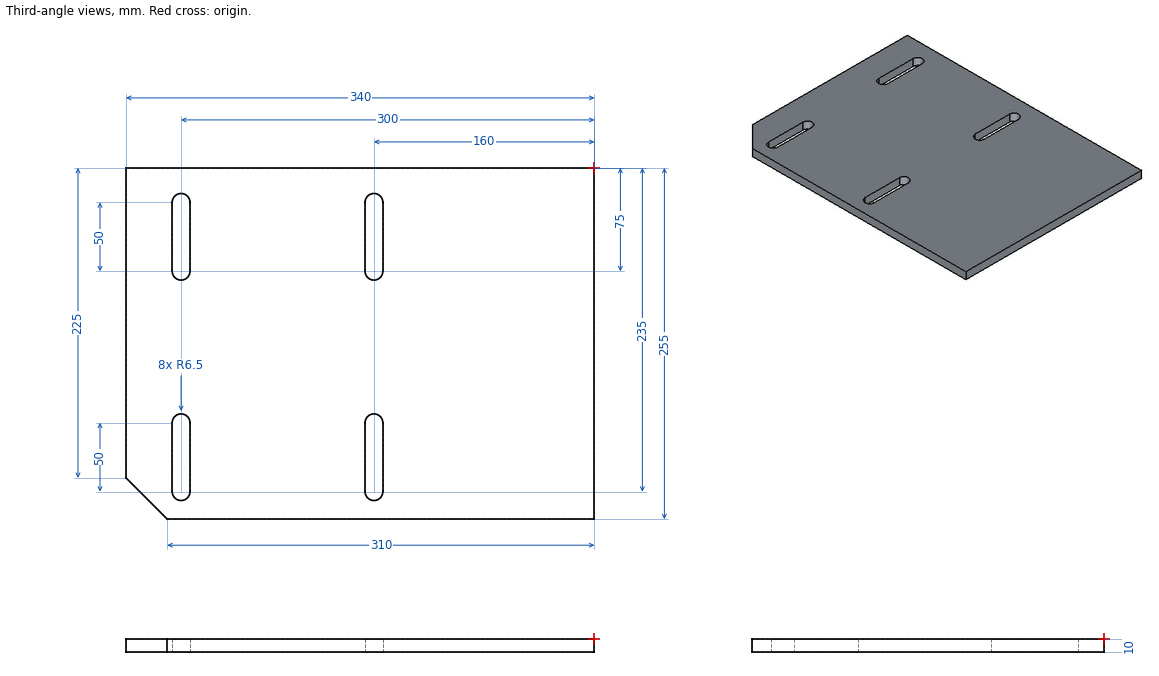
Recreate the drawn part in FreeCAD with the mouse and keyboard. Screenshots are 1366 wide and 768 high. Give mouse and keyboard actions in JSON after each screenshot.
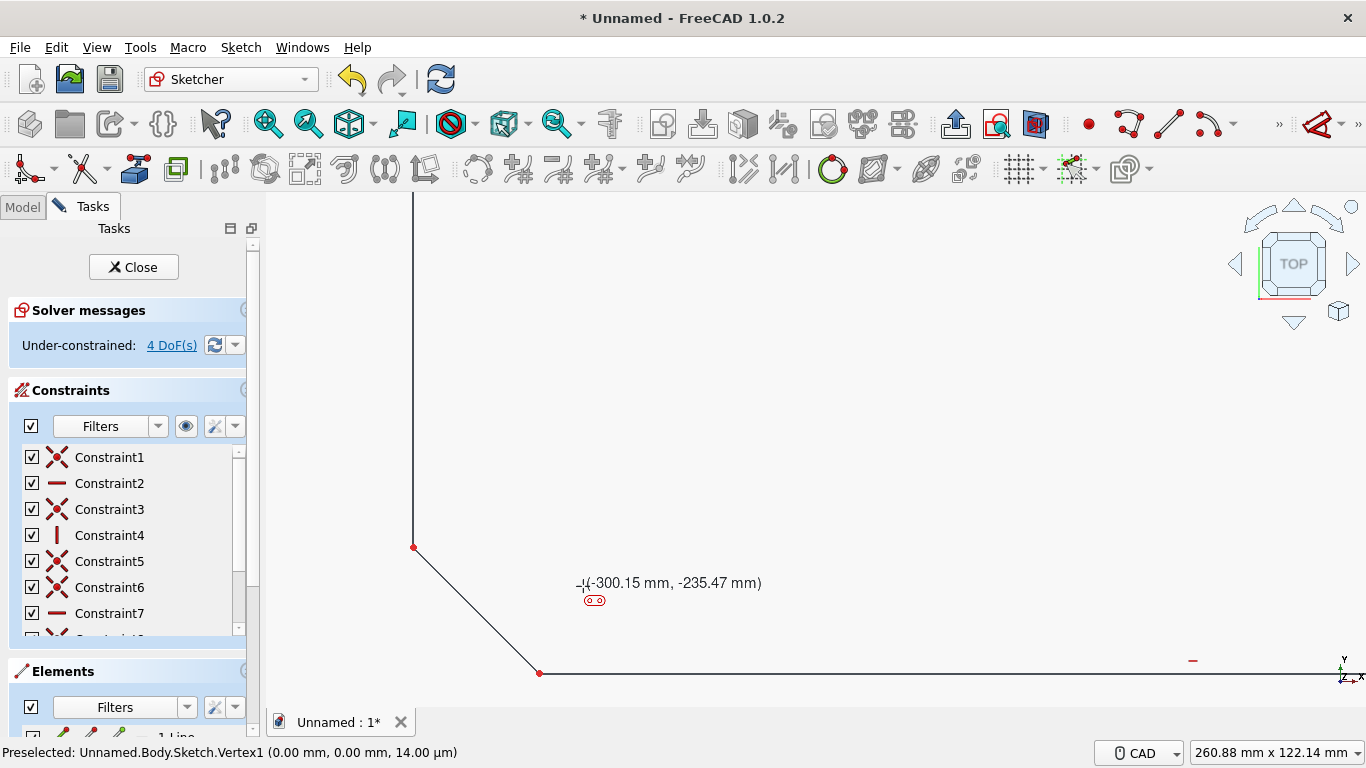
{"action": "left_click", "coordinate": [583, 586]}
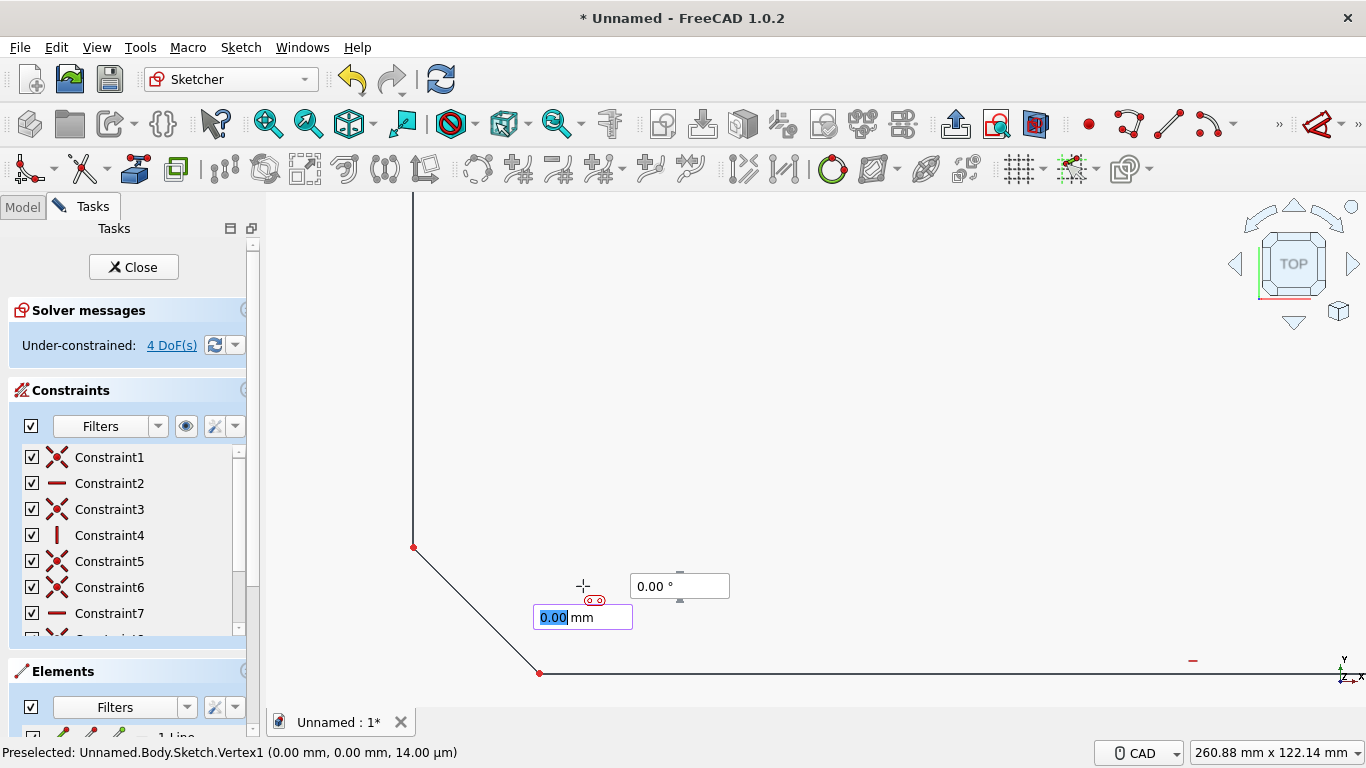
{"action": "left_click", "coordinate": [583, 375]}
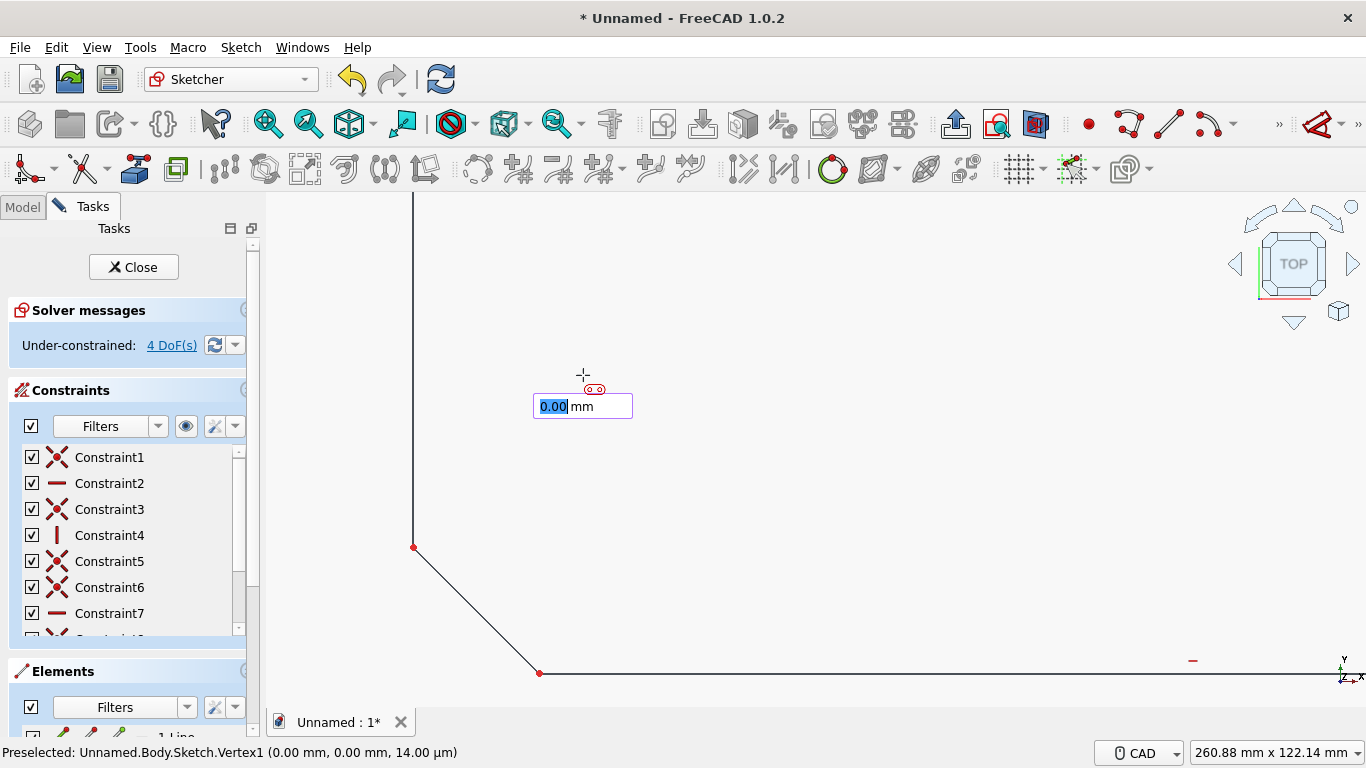
{"action": "left_click", "coordinate": [610, 480]}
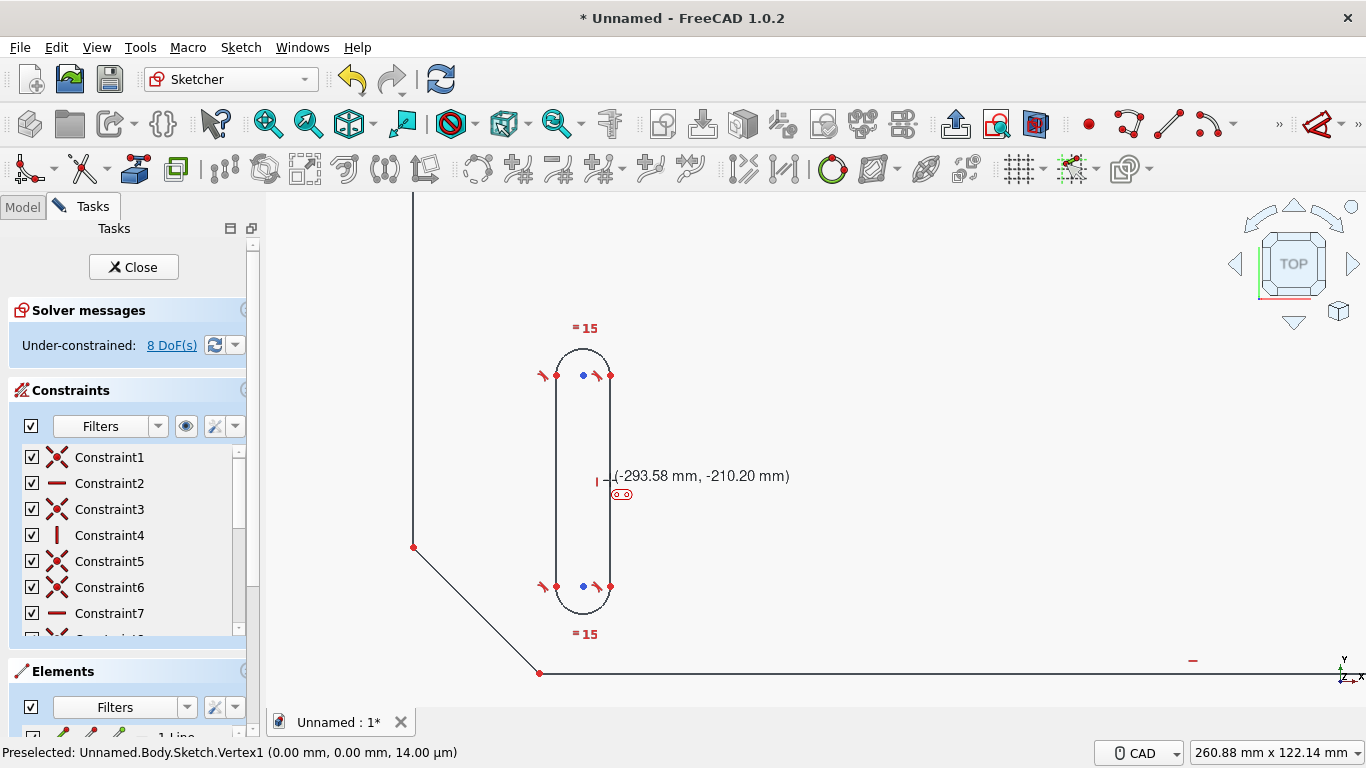
{"action": "left_click", "coordinate": [1173, 586]}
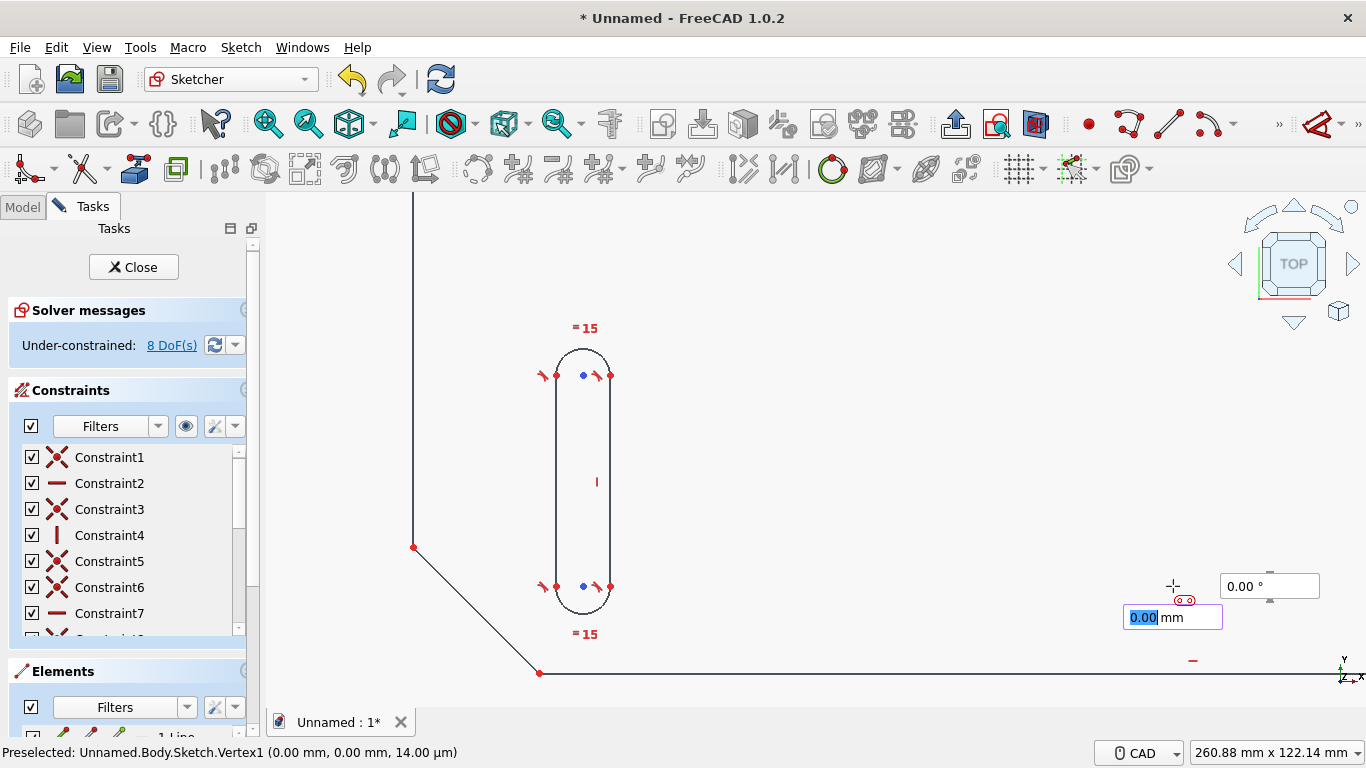
{"action": "left_click", "coordinate": [1173, 375]}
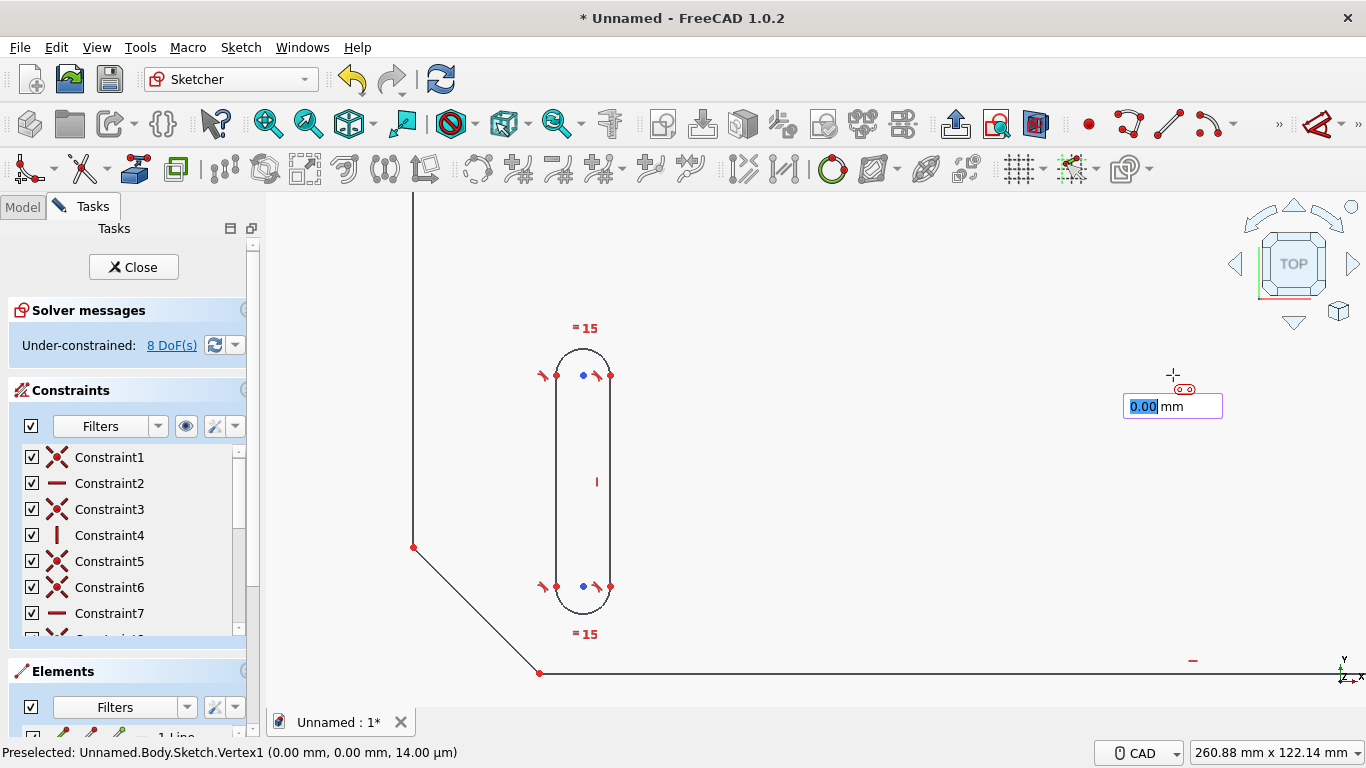
{"action": "left_click", "coordinate": [1201, 480]}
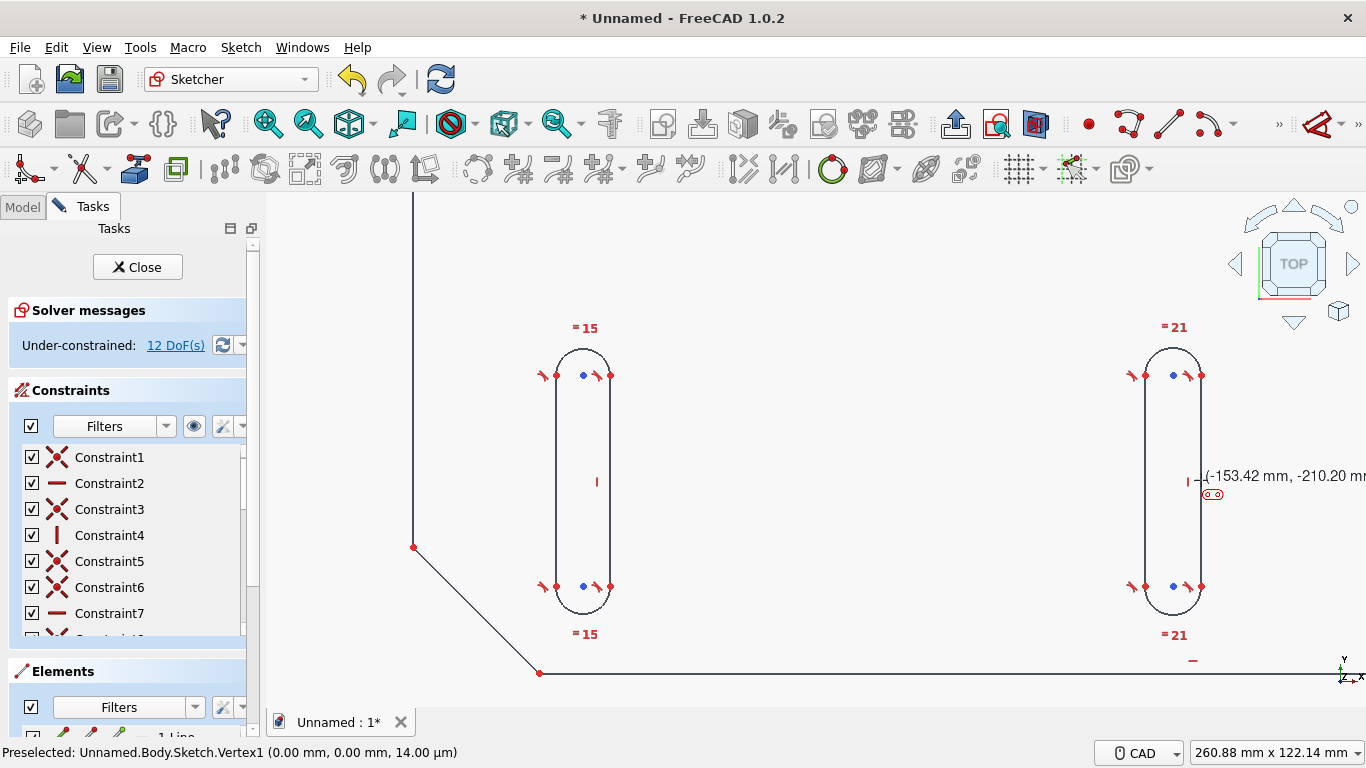
{"action": "scroll", "coordinate": [582, 586], "scroll_direction": "down", "scroll_amount": 6}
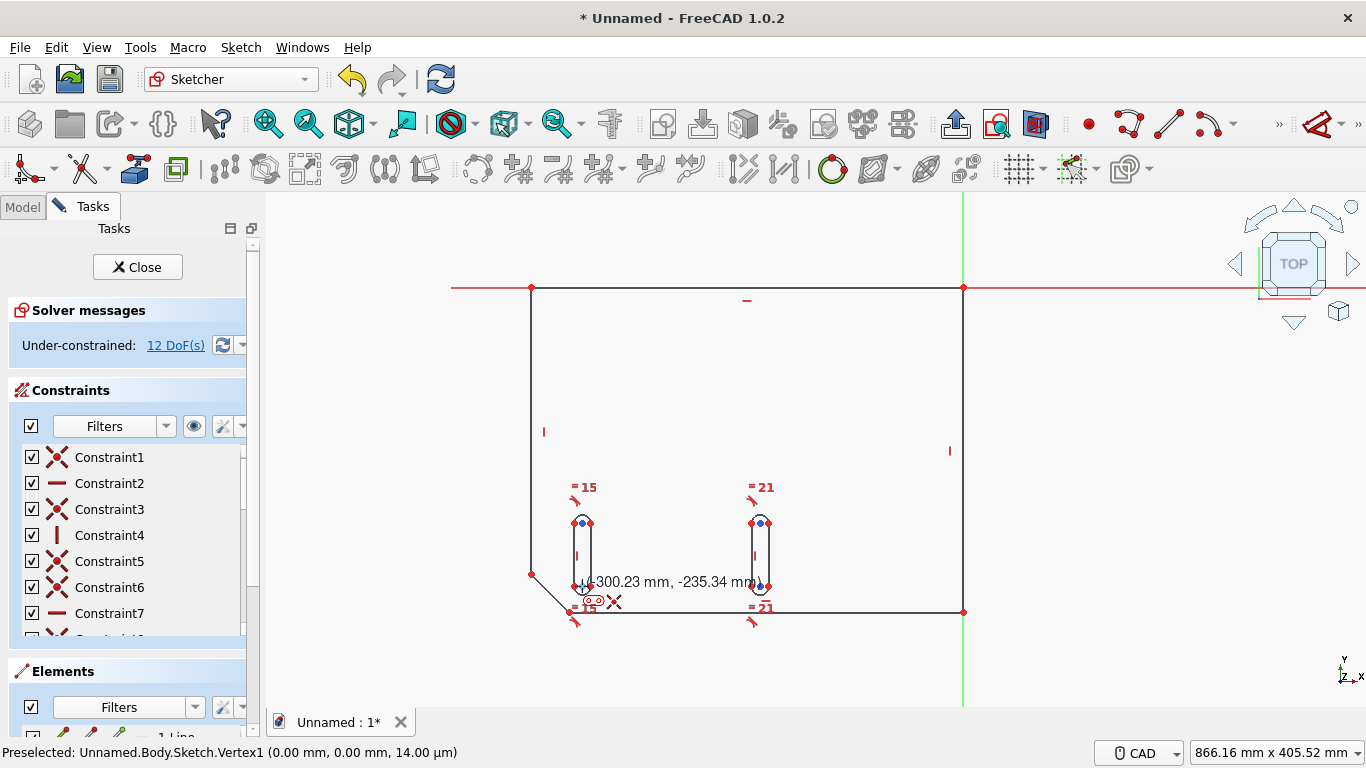
{"action": "scroll", "coordinate": [582, 383], "scroll_direction": "up", "scroll_amount": 6}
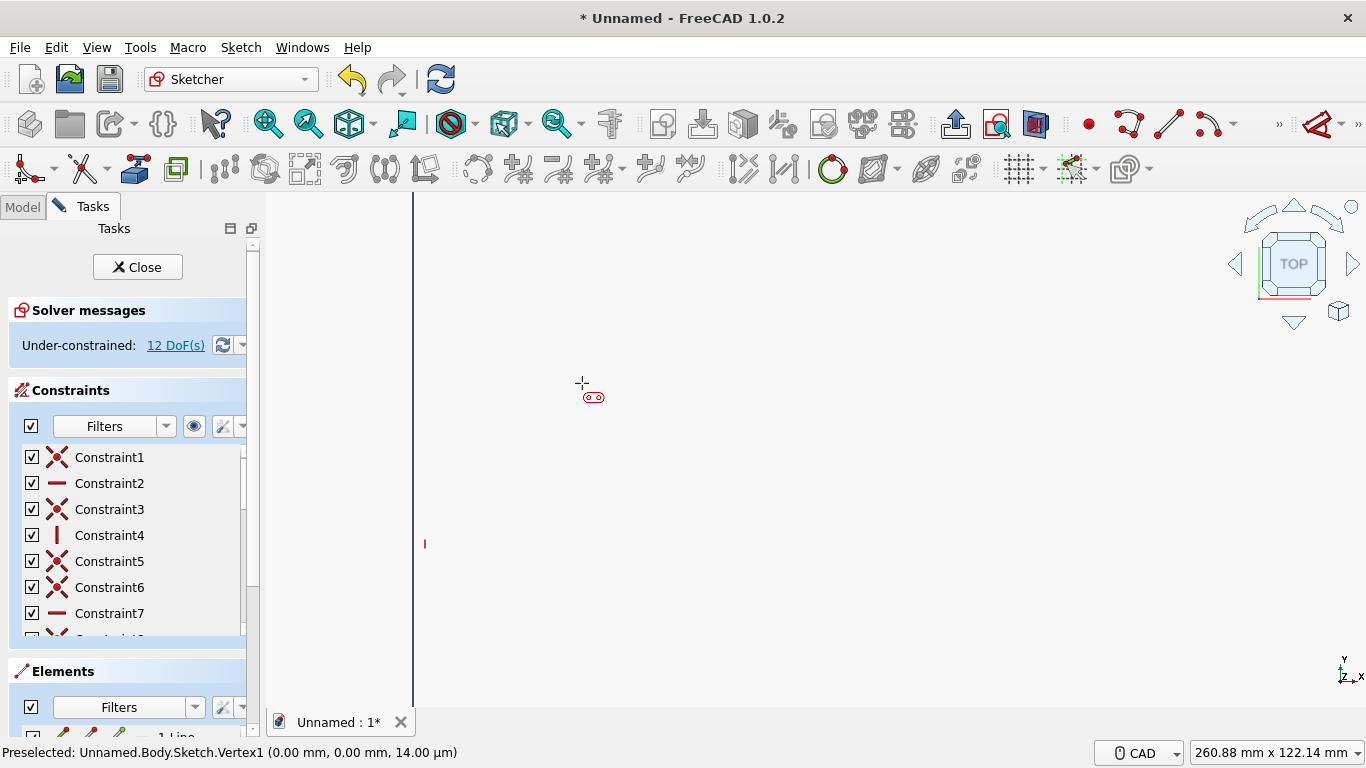
{"action": "left_click", "coordinate": [583, 383]}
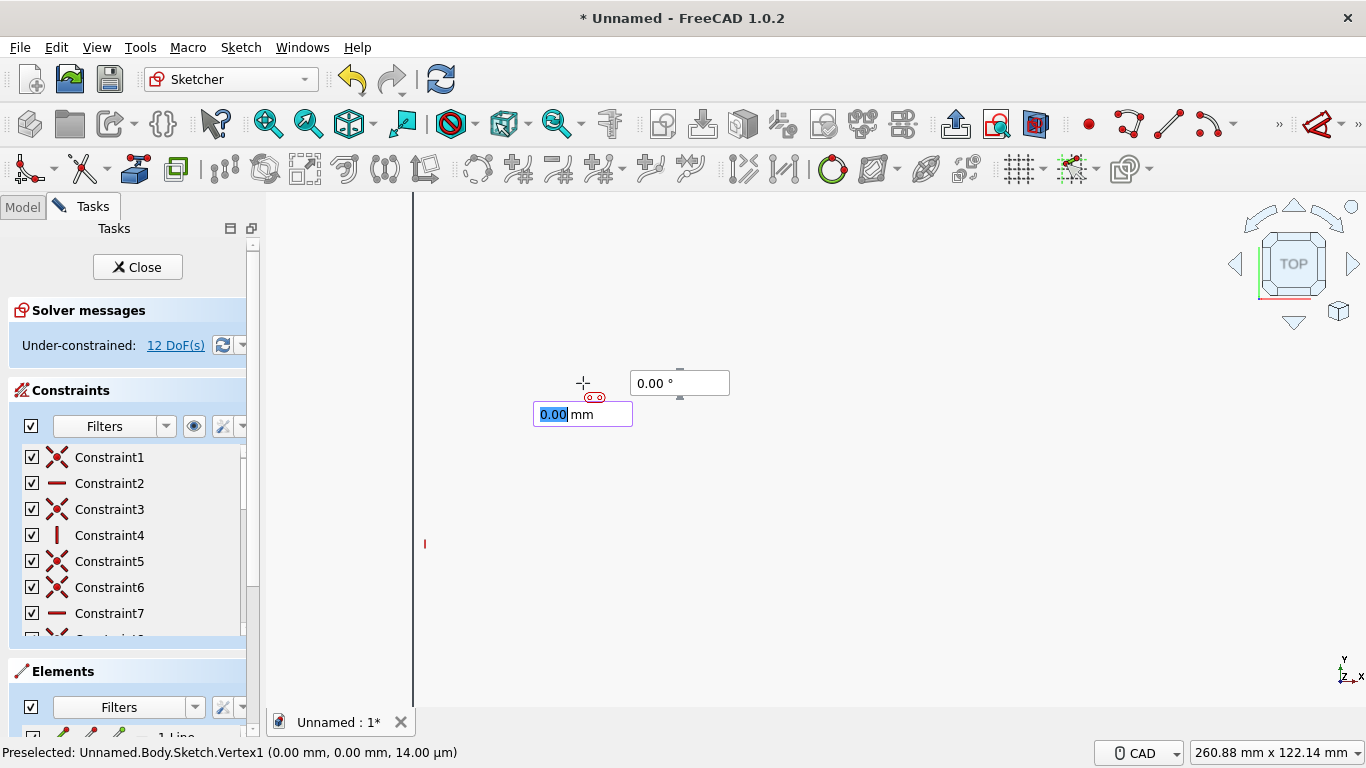
{"action": "scroll", "coordinate": [582, 383], "scroll_direction": "down", "scroll_amount": 6}